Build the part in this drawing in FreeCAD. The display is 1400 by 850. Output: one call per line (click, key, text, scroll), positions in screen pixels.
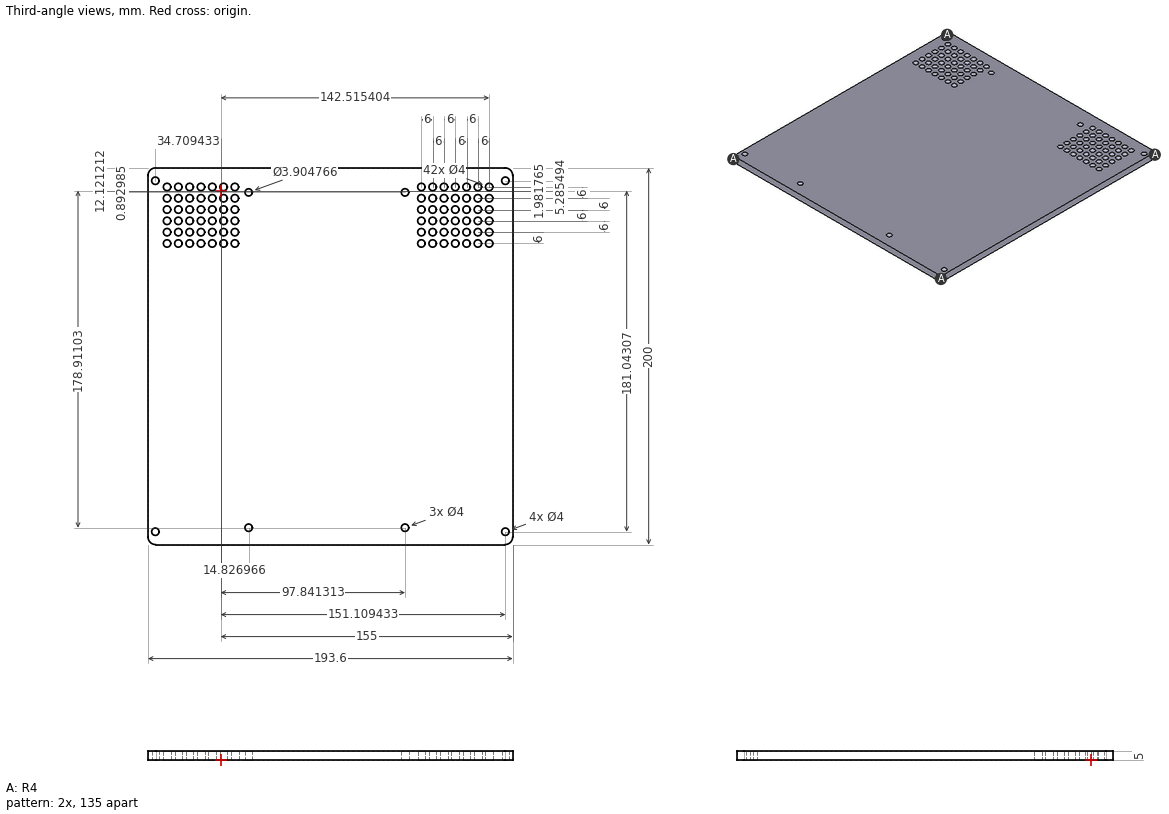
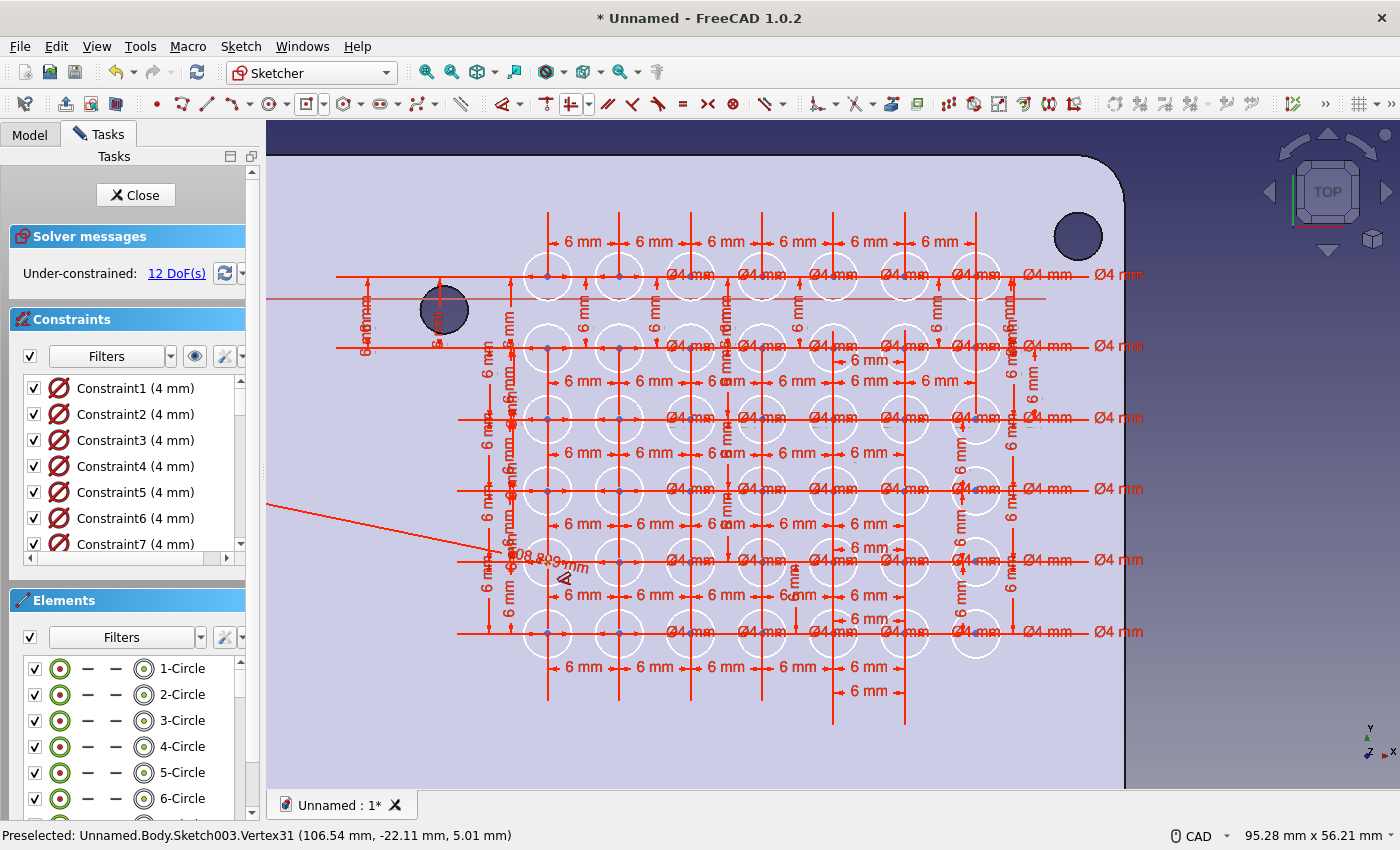
click(548, 634)
click(490, 623)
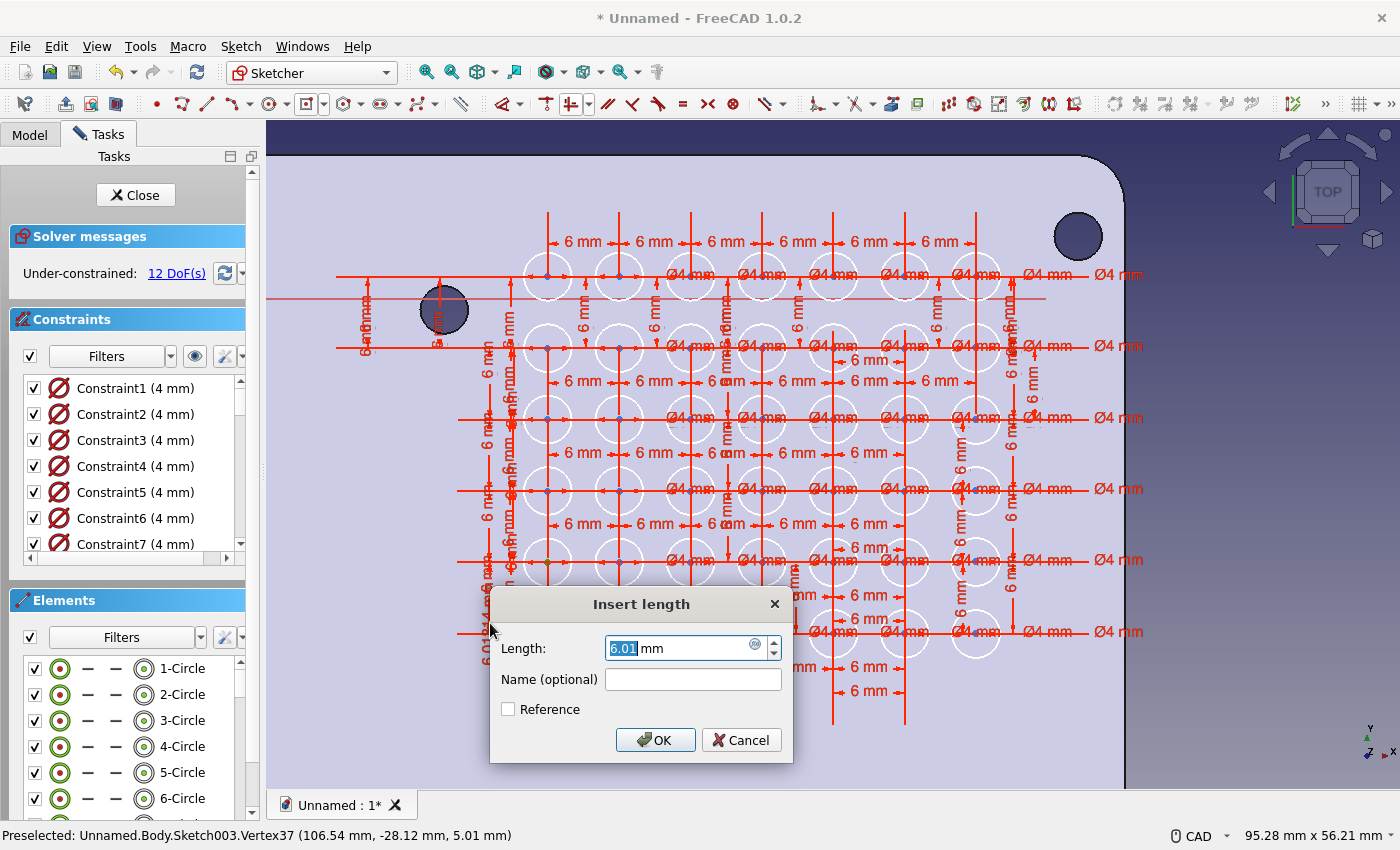
text(6)
key(Return)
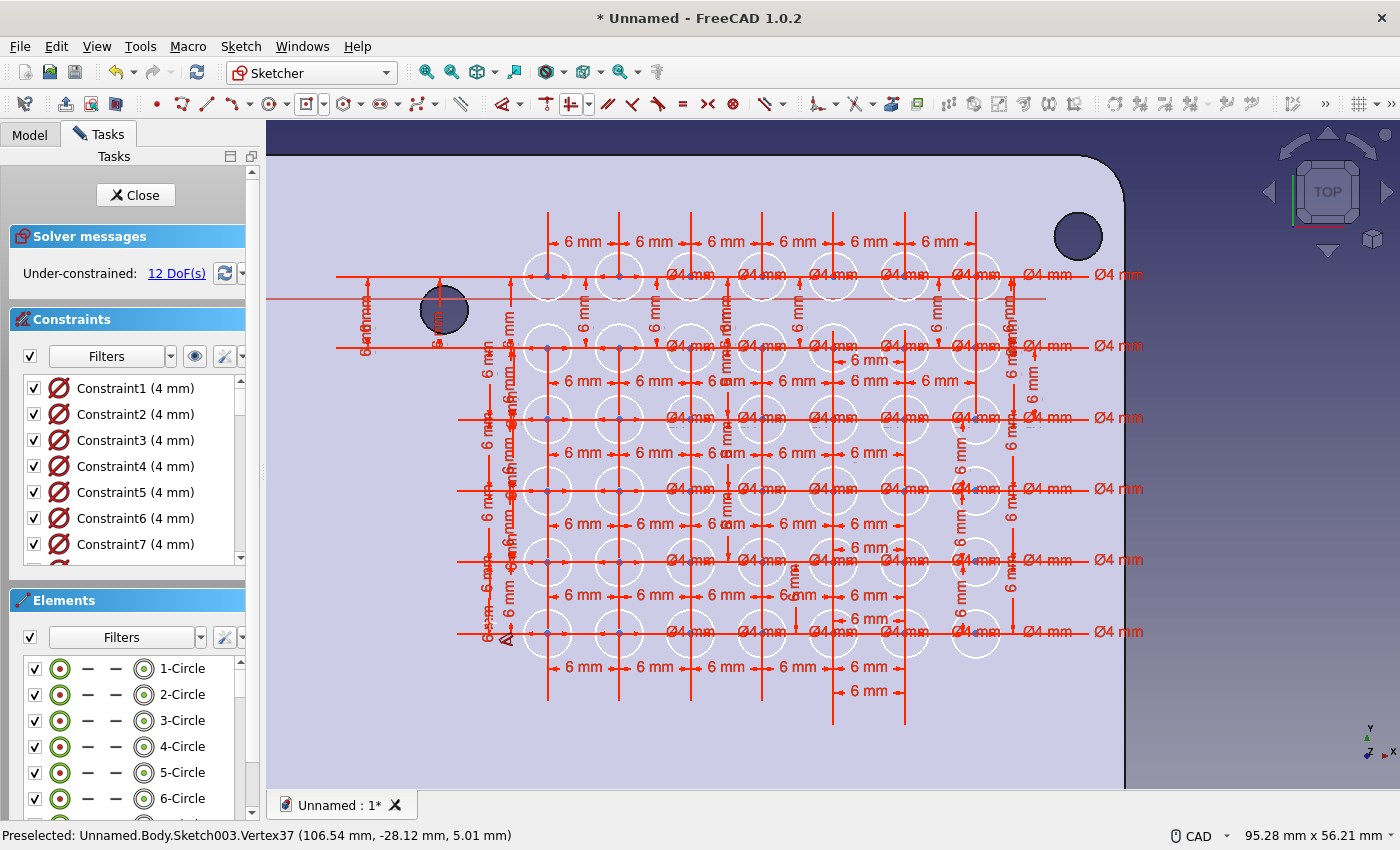
click(905, 348)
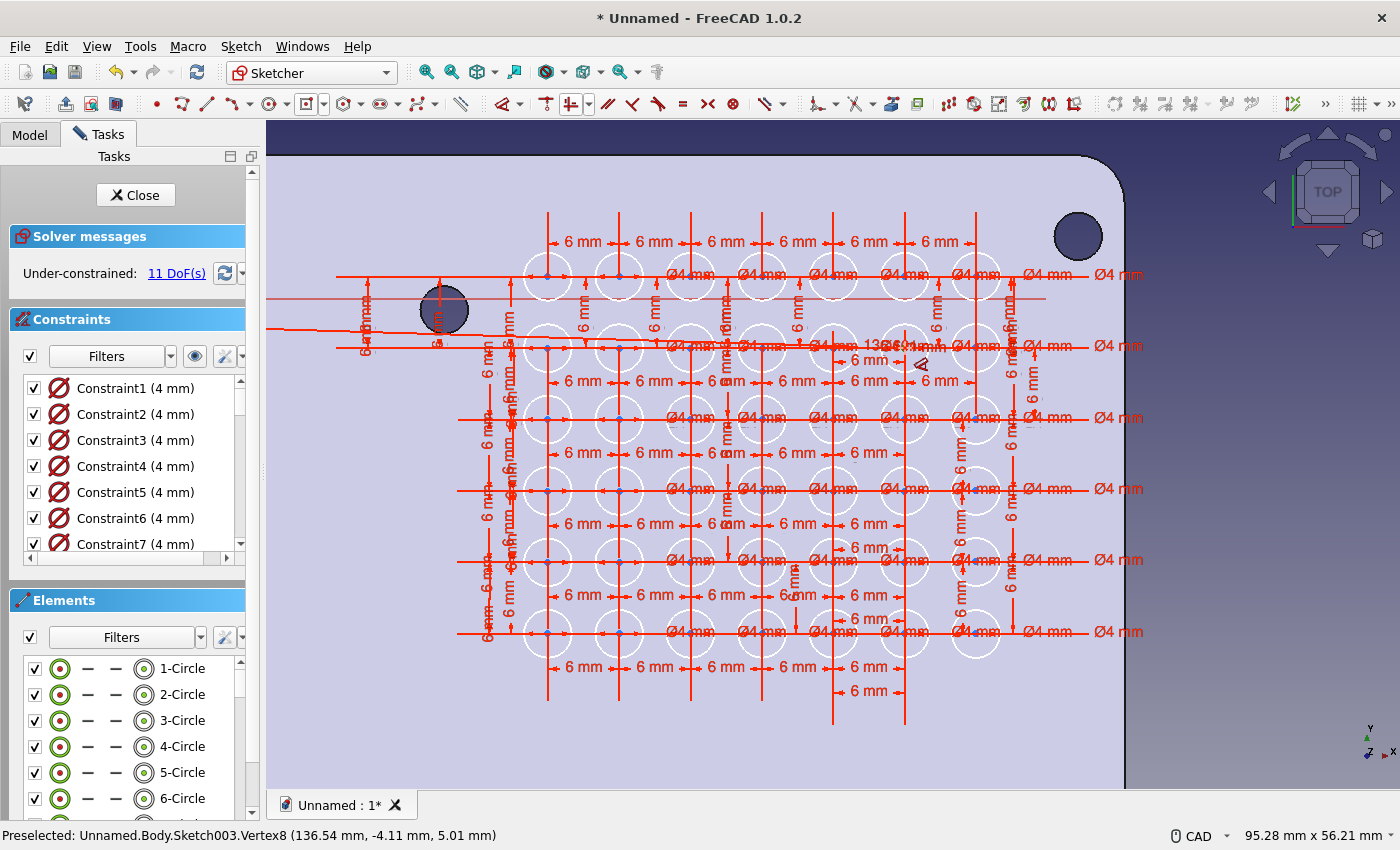
click(976, 348)
click(940, 406)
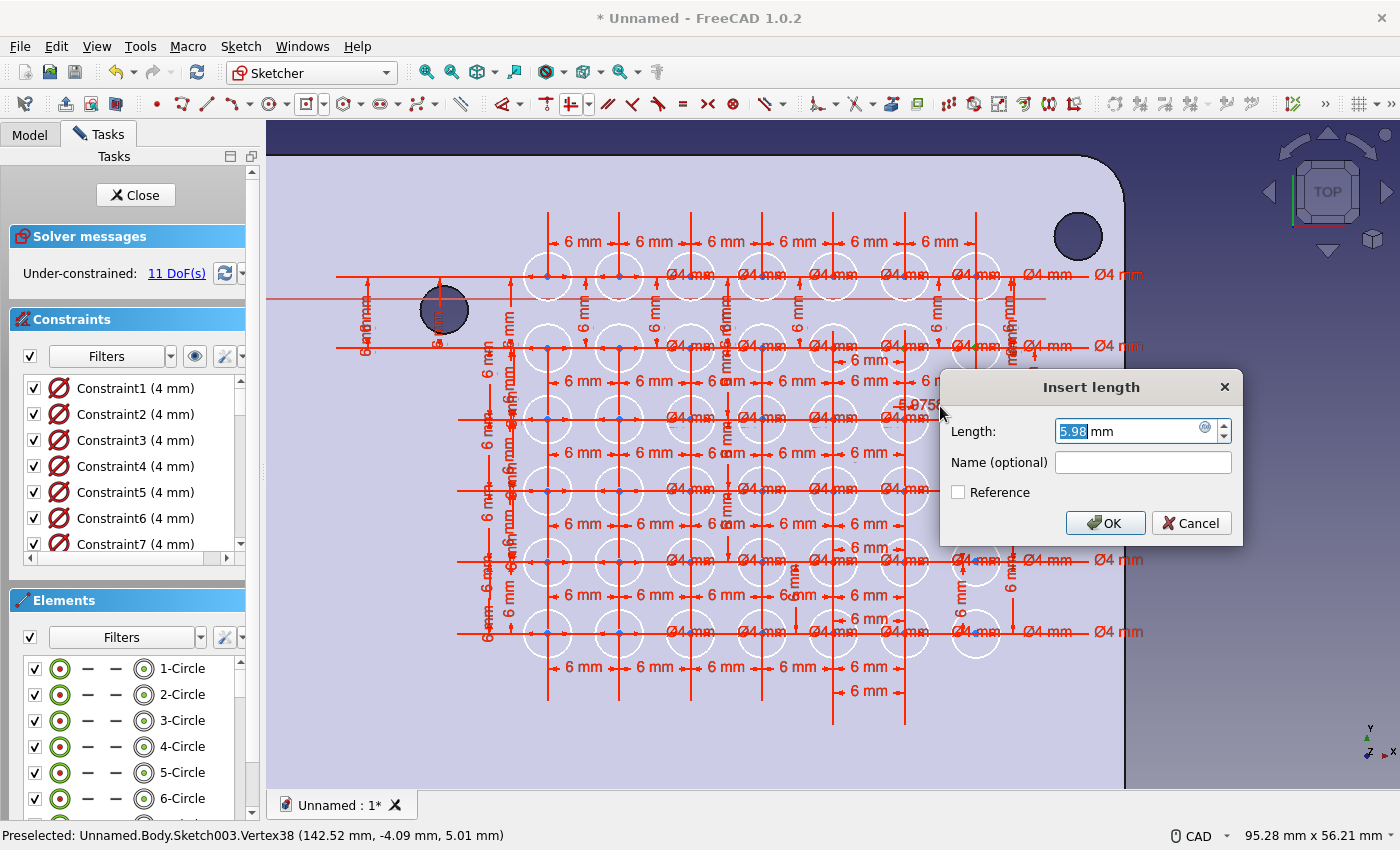
text(6)
key(Return)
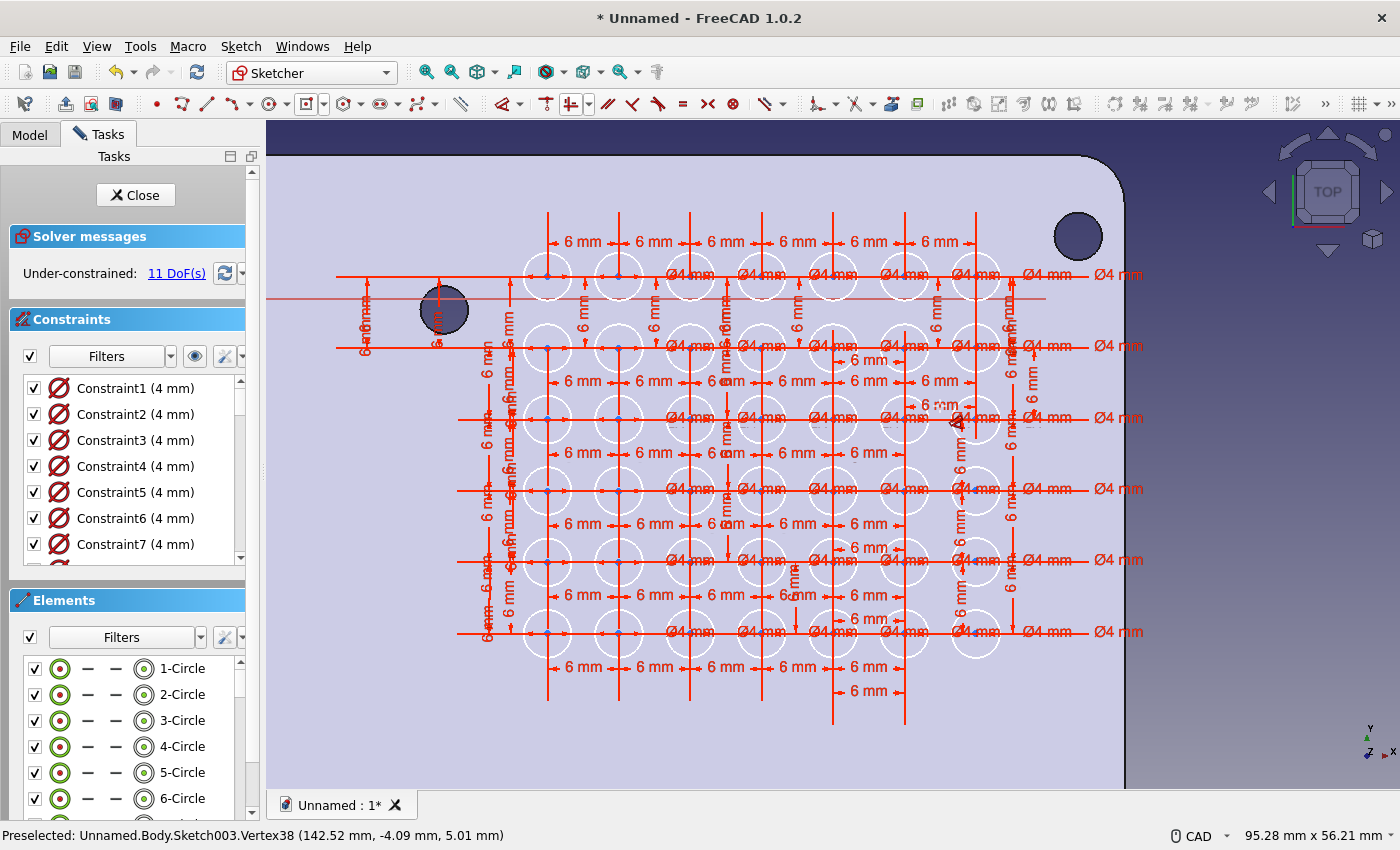
click(976, 277)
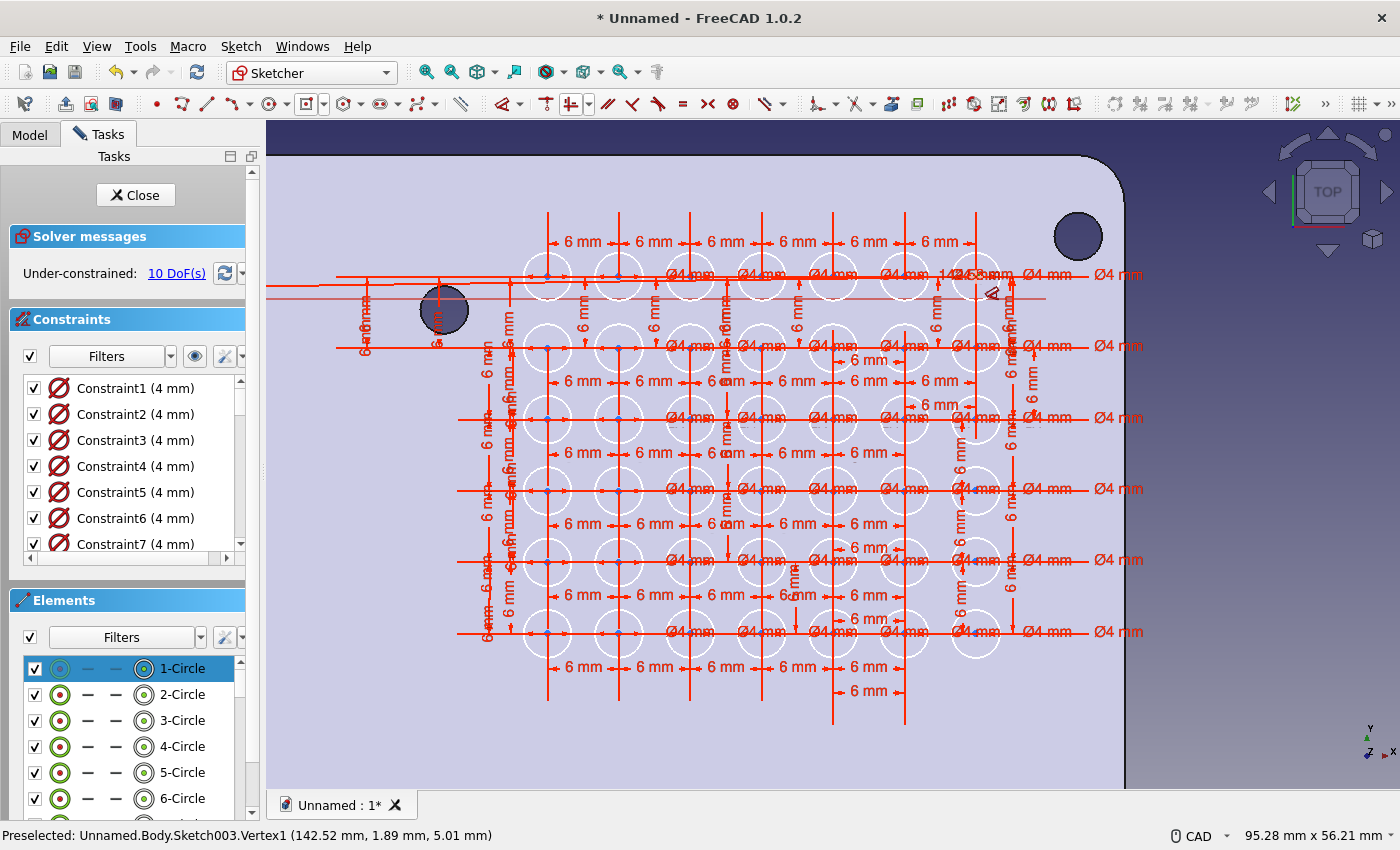
click(976, 348)
click(1082, 312)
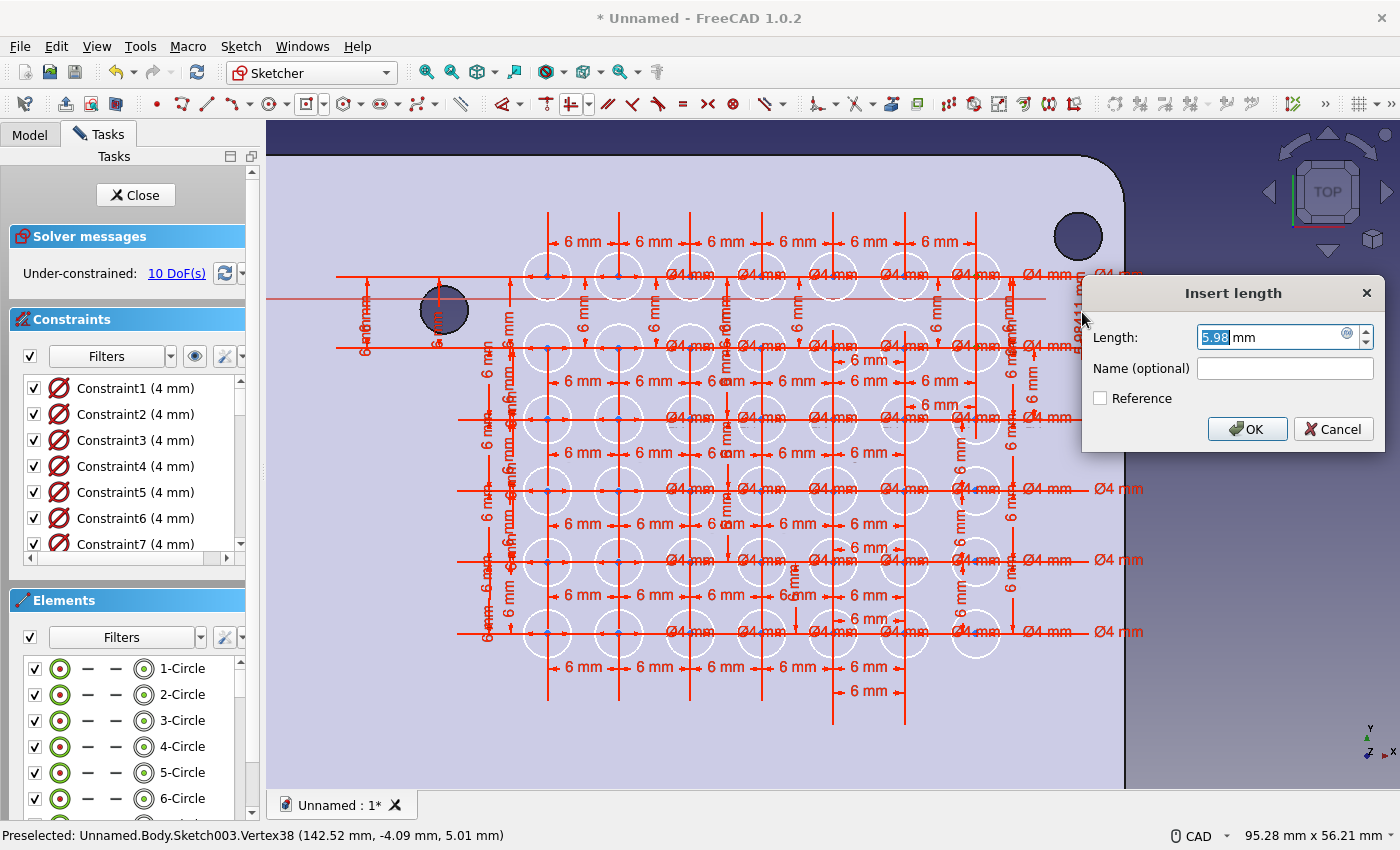
text(6)
key(Return)